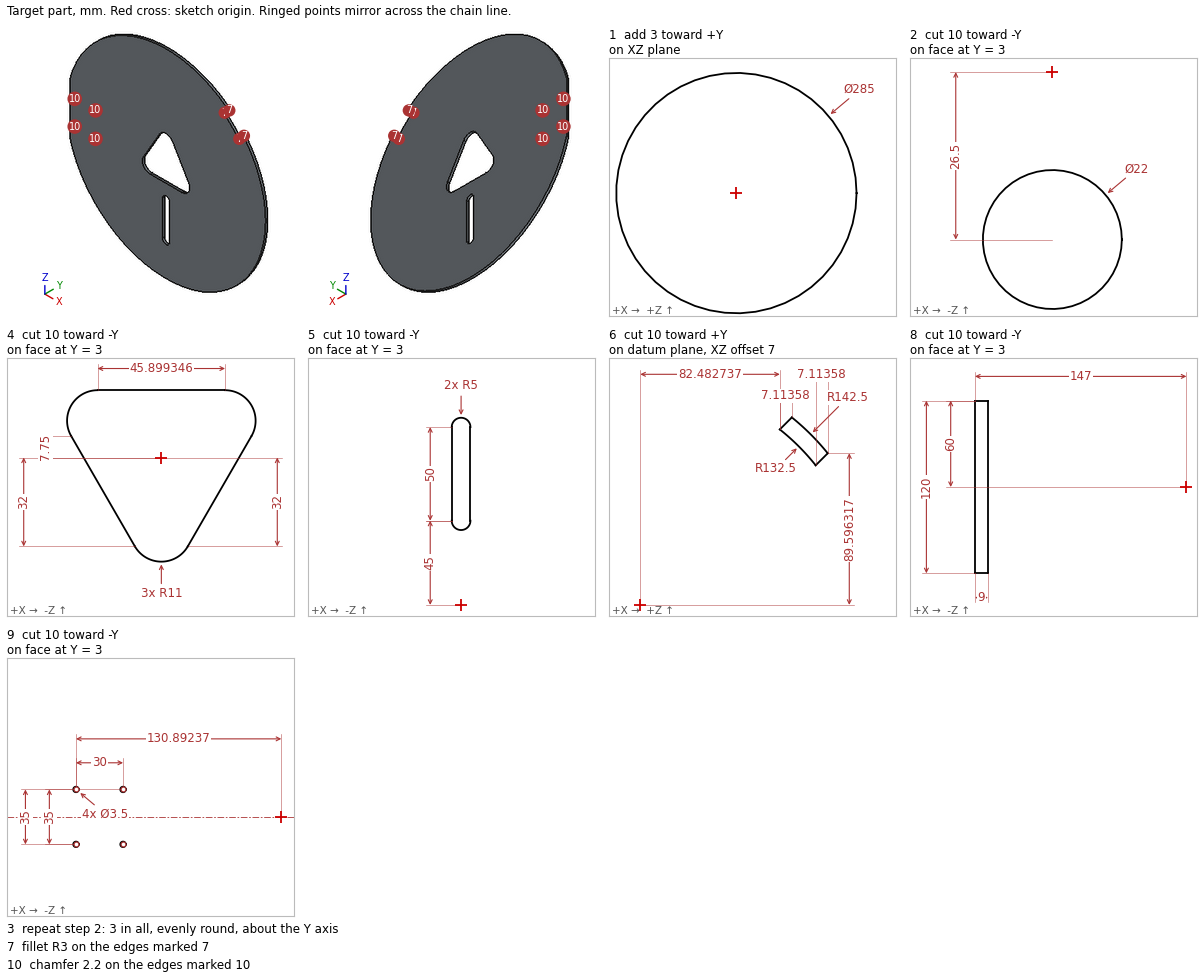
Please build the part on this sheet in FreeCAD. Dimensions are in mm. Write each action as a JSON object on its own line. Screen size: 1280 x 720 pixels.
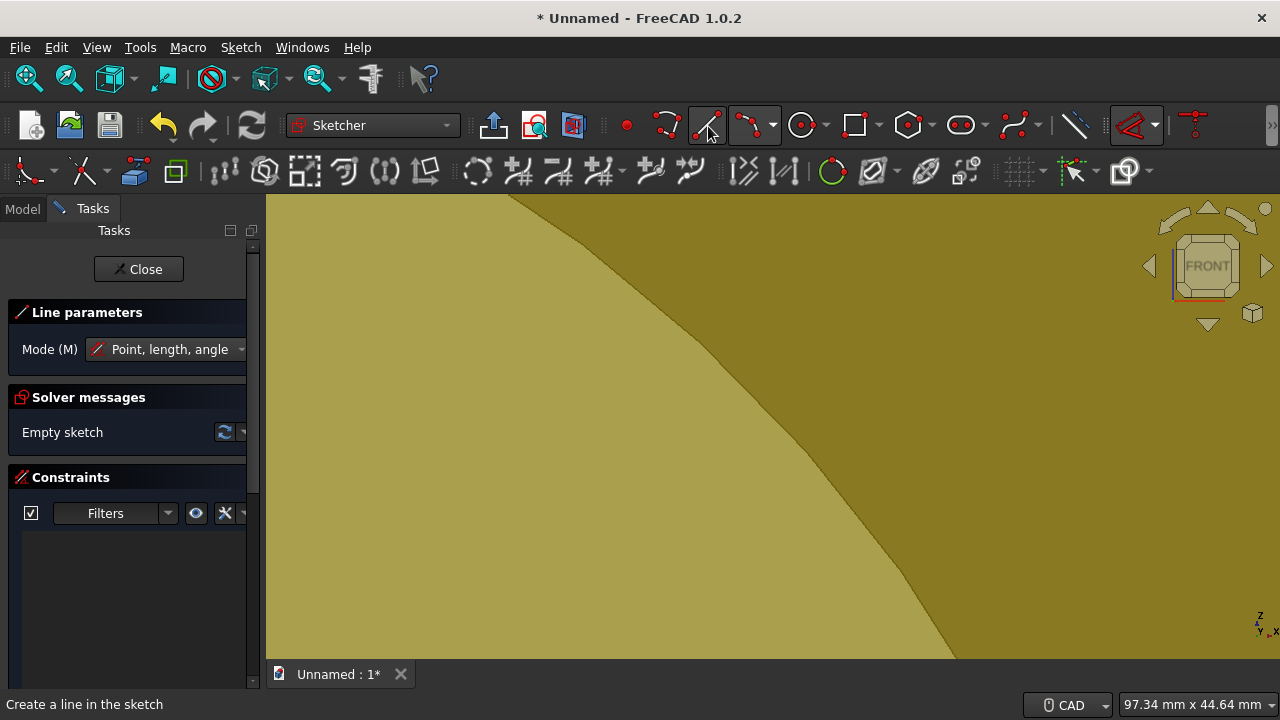
{"action": "left_click", "coordinate": [551, 352]}
{"action": "left_click", "coordinate": [625, 277]}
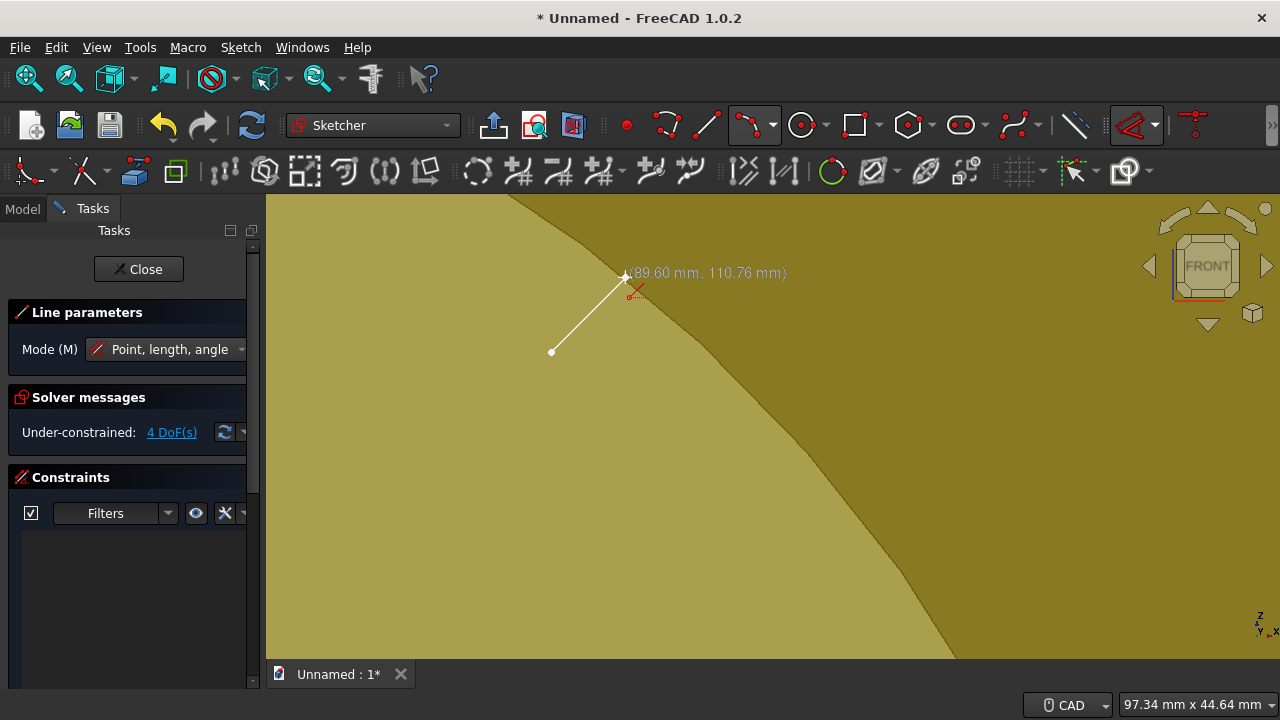
{"action": "left_click", "coordinate": [846, 498]}
{"action": "left_click", "coordinate": [772, 573]}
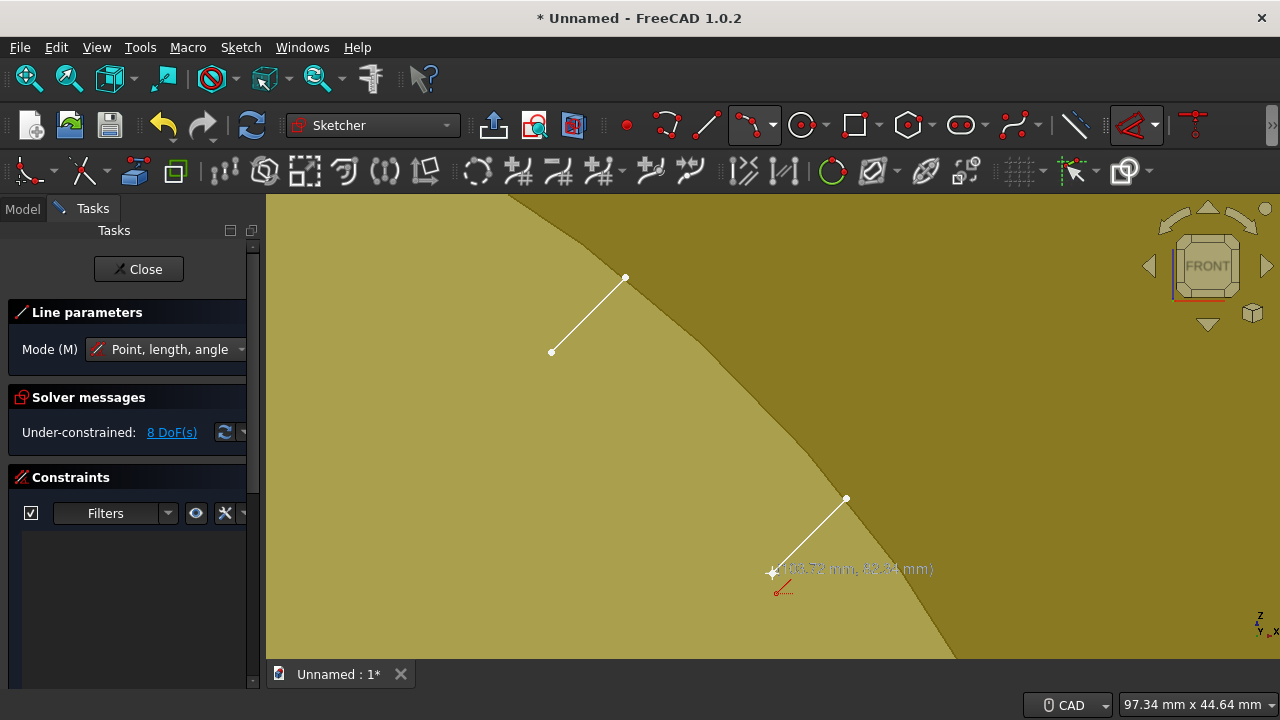
{"action": "left_click", "coordinate": [748, 126]}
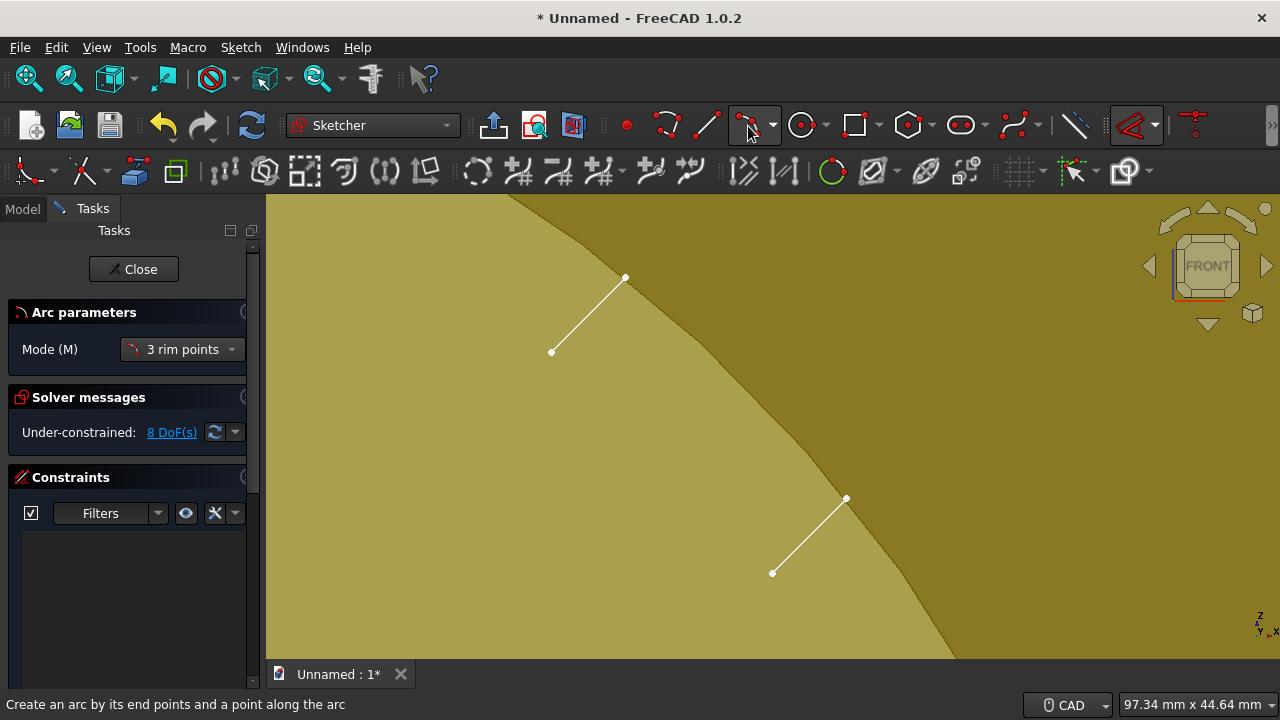
{"action": "left_click", "coordinate": [625, 278]}
{"action": "left_click", "coordinate": [846, 499]}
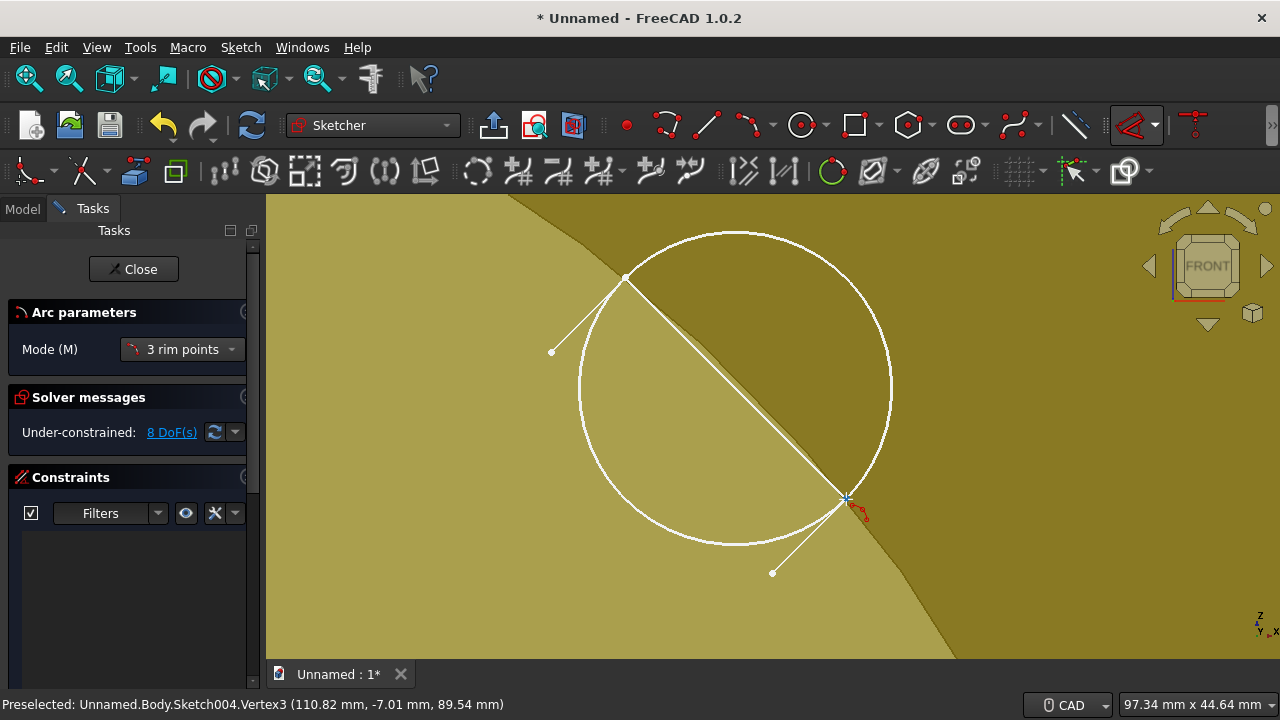
{"action": "scroll", "coordinate": [741, 382], "scroll_direction": "up", "scroll_amount": 4}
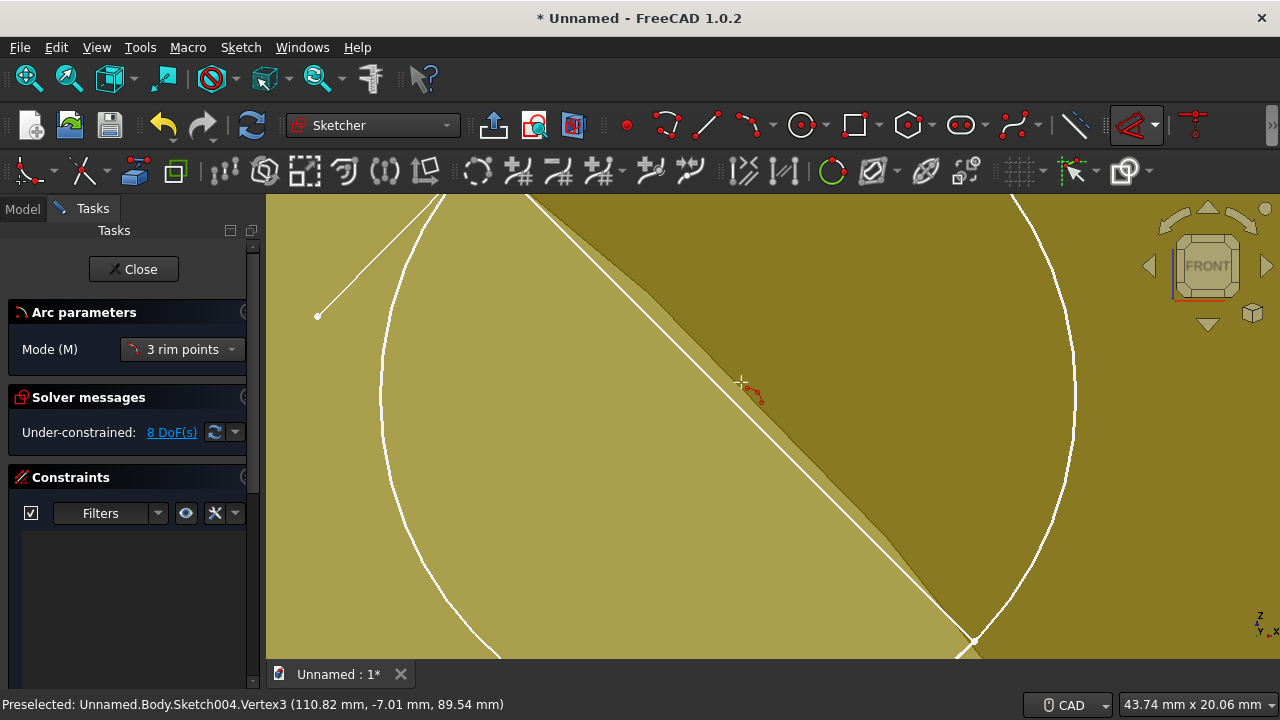
{"action": "left_click", "coordinate": [741, 382]}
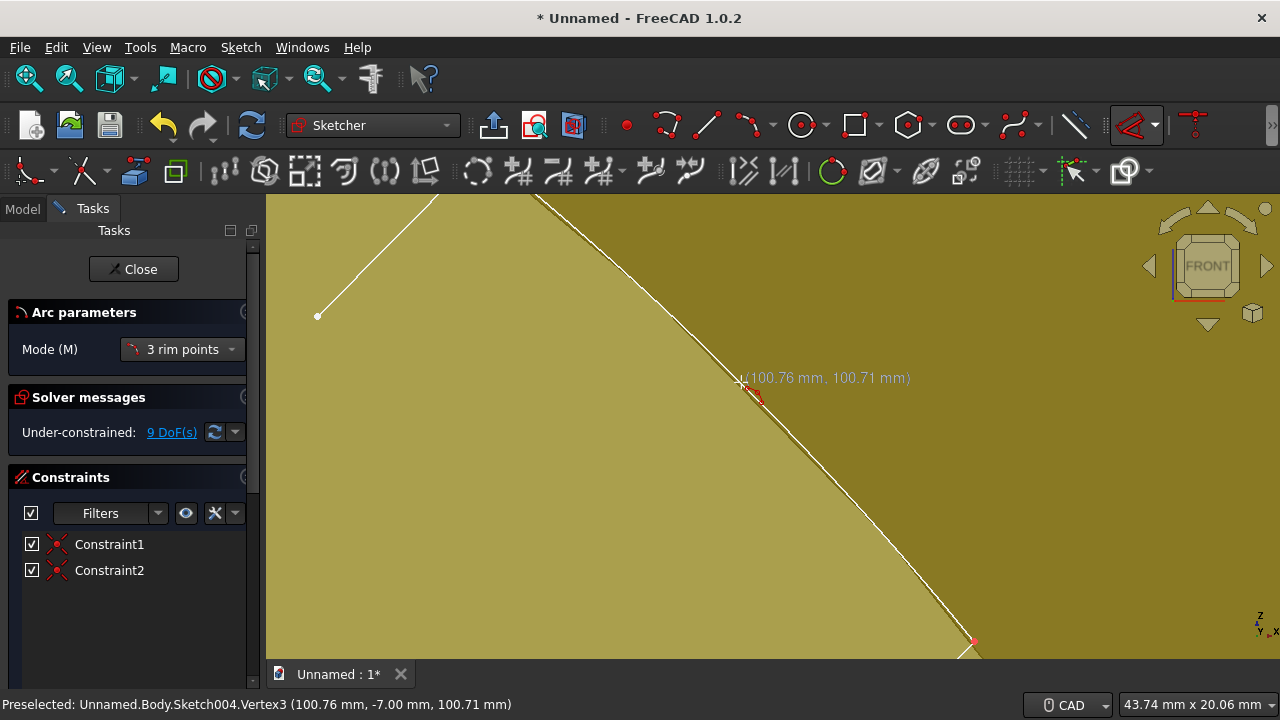
{"action": "scroll", "coordinate": [753, 385], "scroll_direction": "down", "scroll_amount": 4}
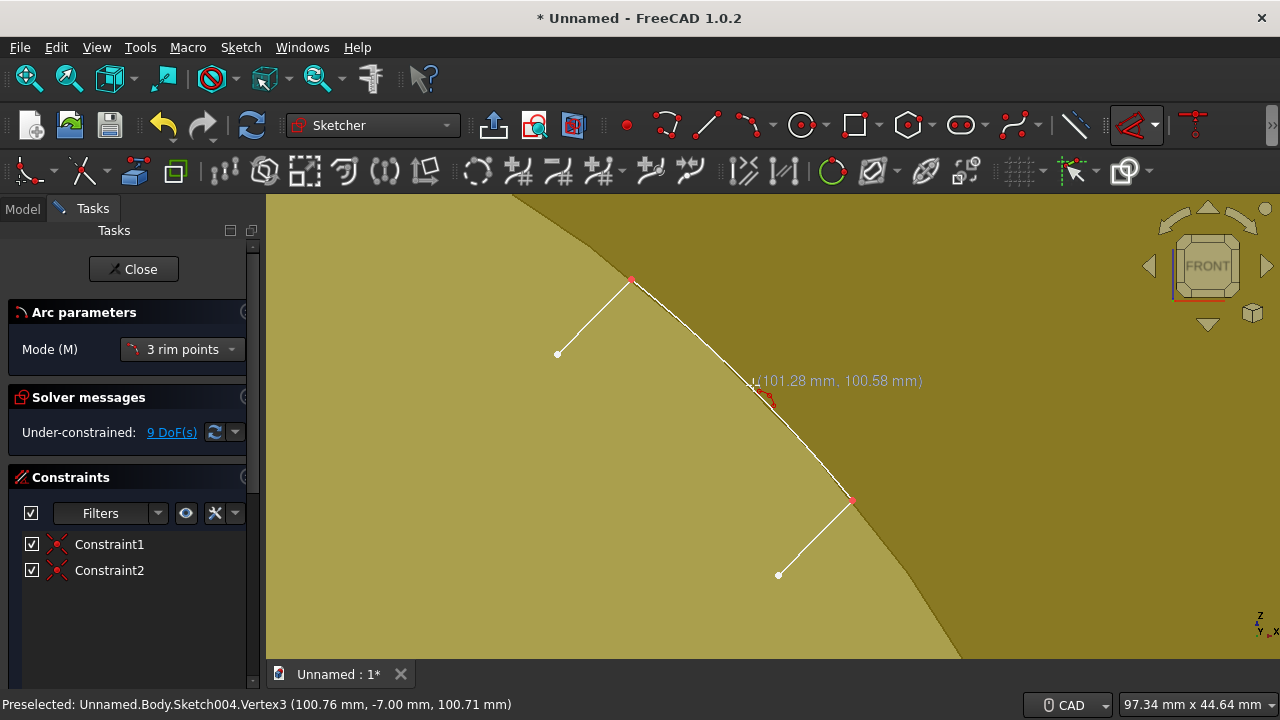
{"action": "left_click", "coordinate": [779, 576]}
{"action": "left_click", "coordinate": [558, 355]}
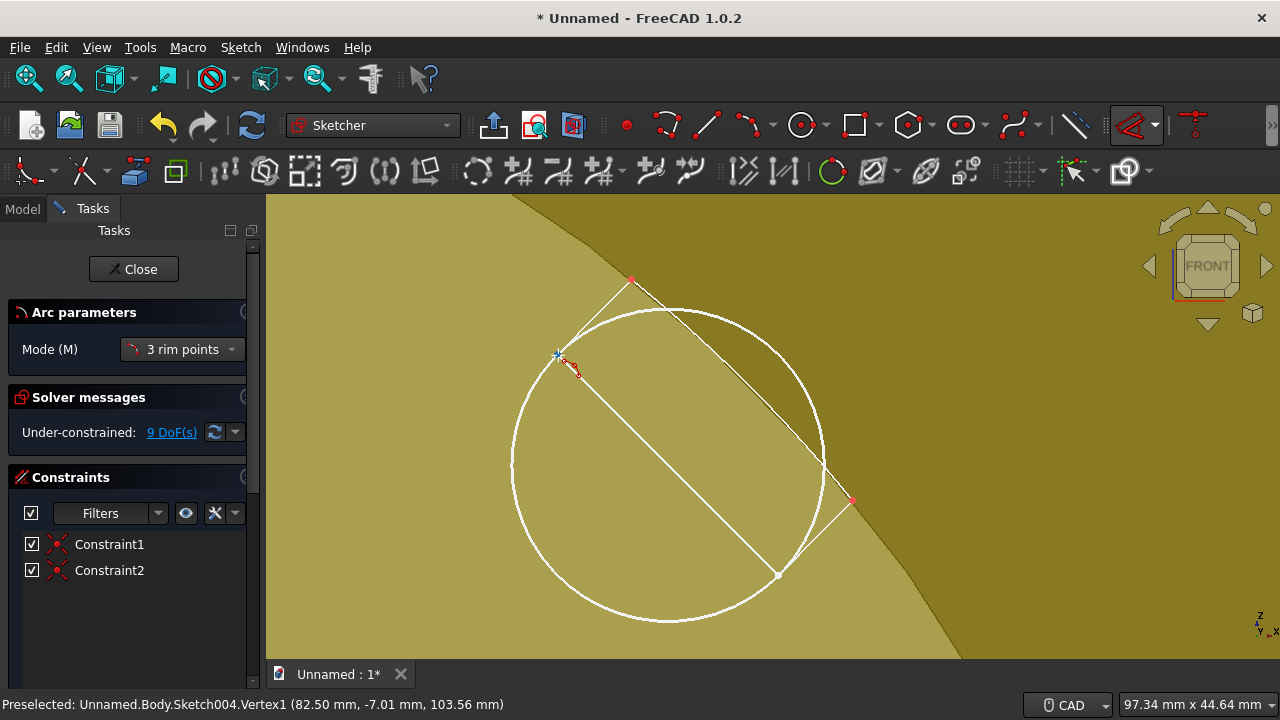
{"action": "scroll", "coordinate": [674, 457], "scroll_direction": "up", "scroll_amount": 3}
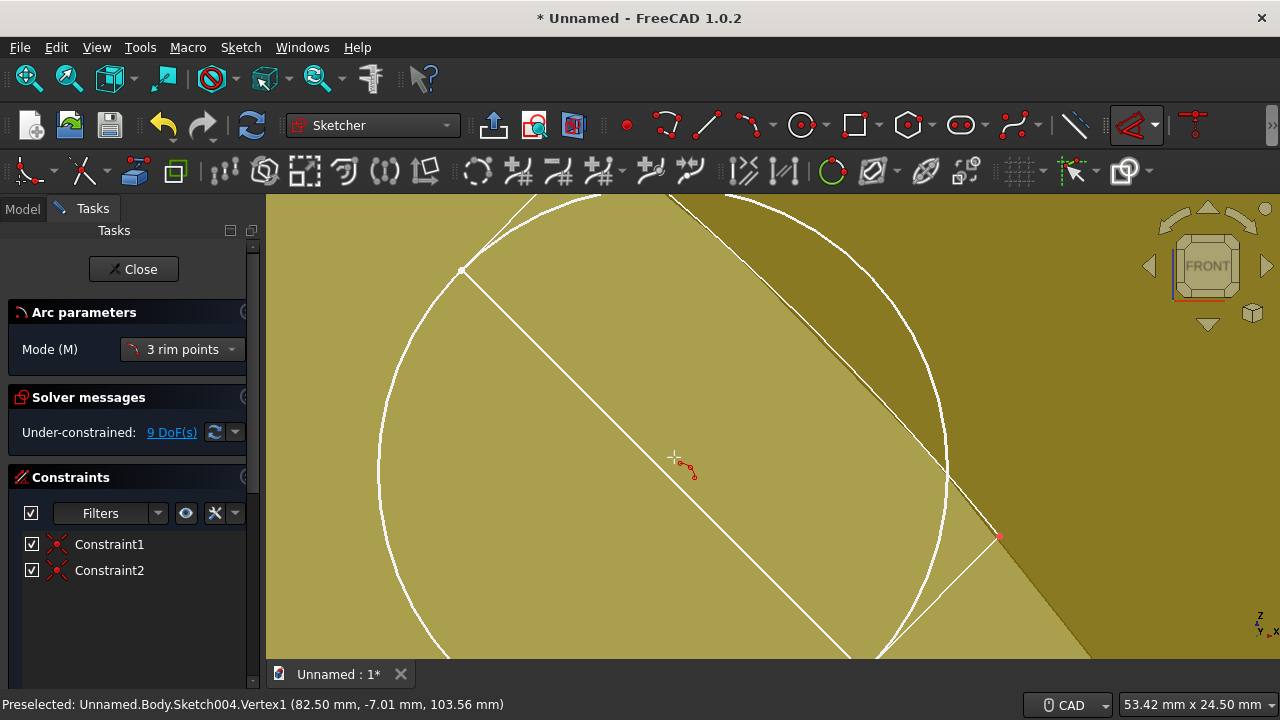
{"action": "left_click", "coordinate": [674, 457]}
{"action": "key", "text": "Escape"}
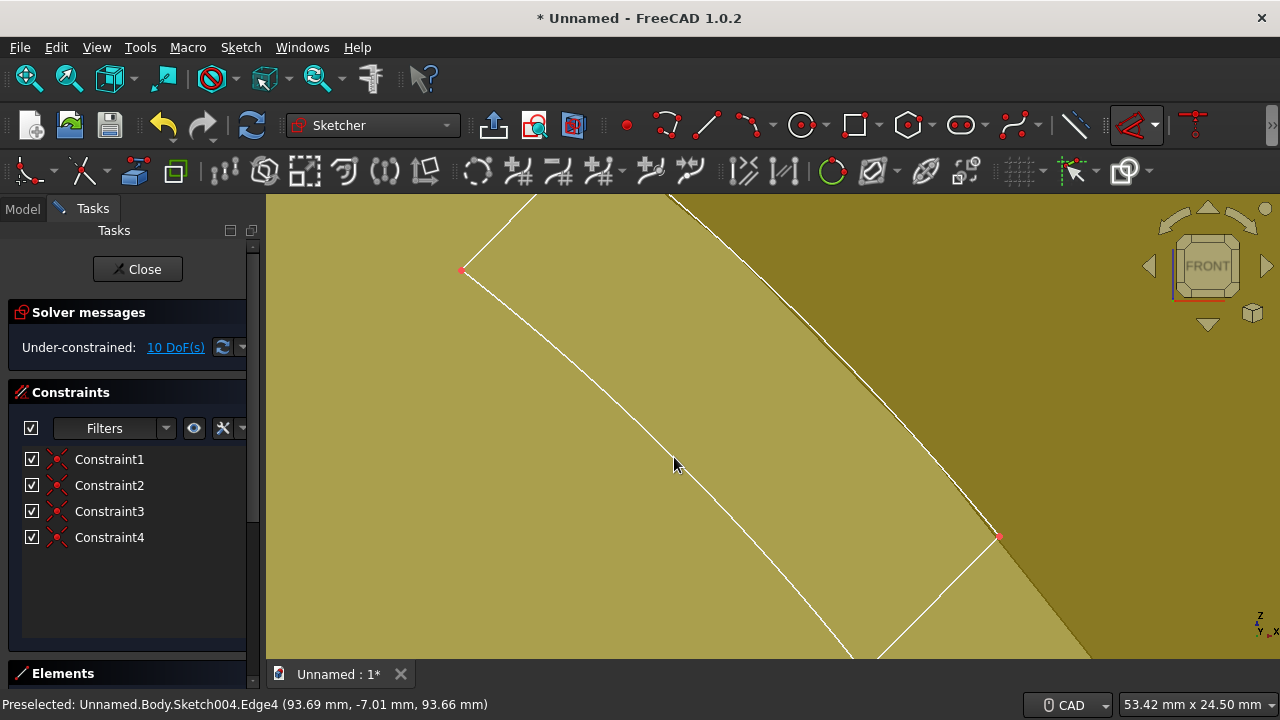
{"action": "left_click", "coordinate": [887, 407]}